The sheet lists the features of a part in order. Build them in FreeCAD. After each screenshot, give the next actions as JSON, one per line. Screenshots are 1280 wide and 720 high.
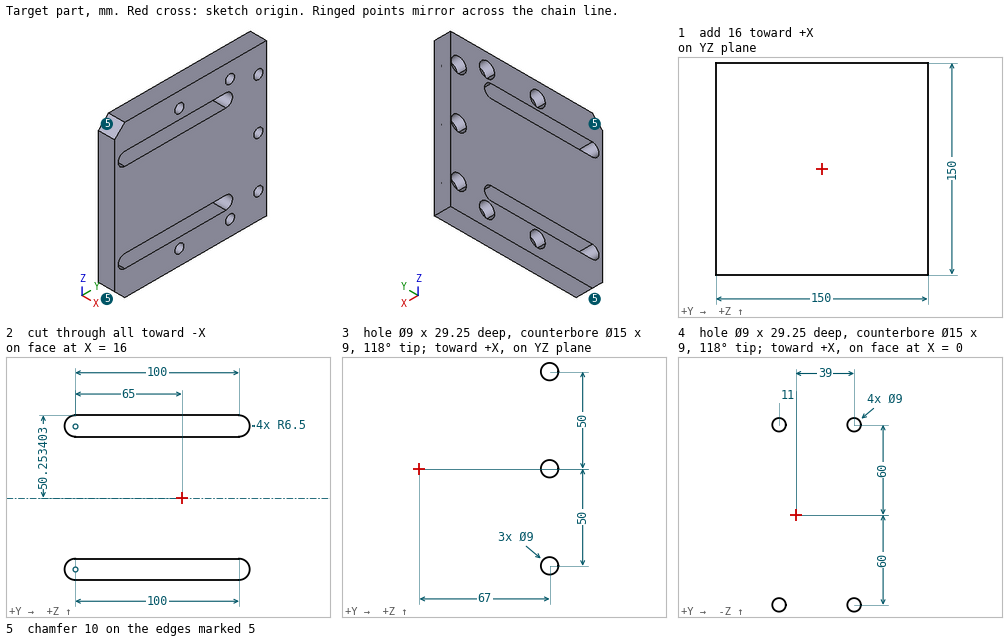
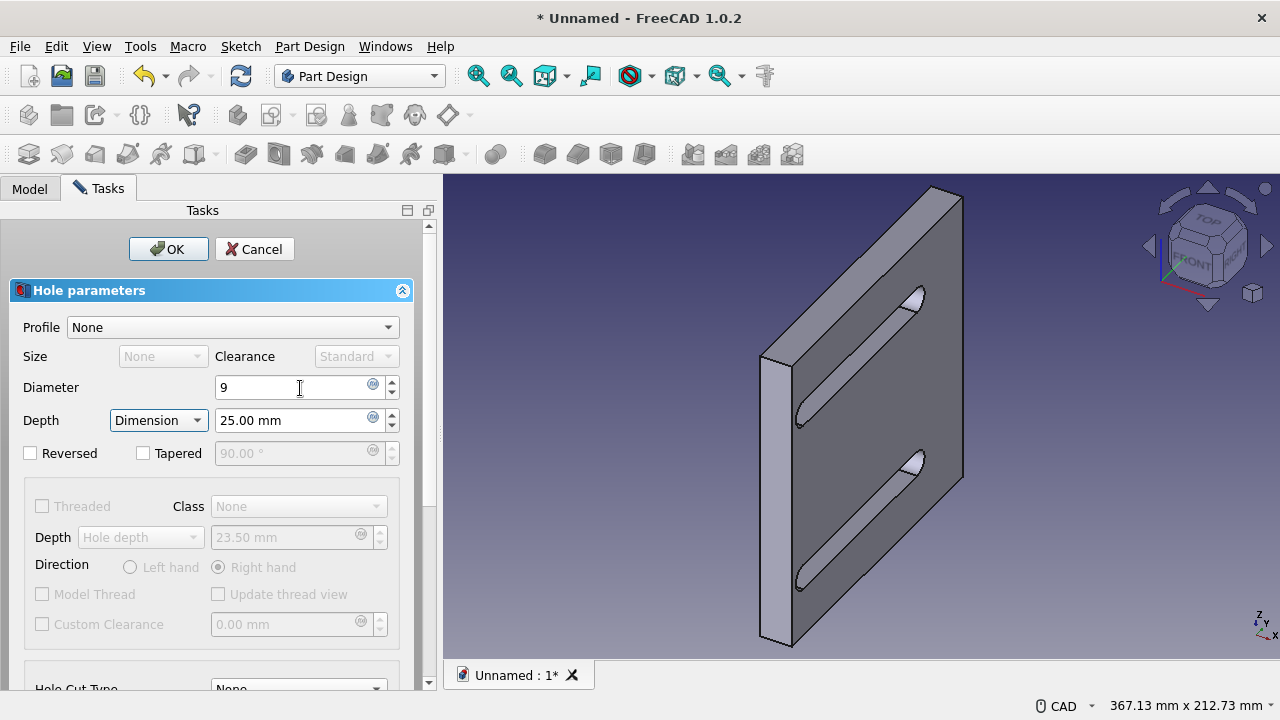
{"action": "triple_click", "coordinate": [300, 420]}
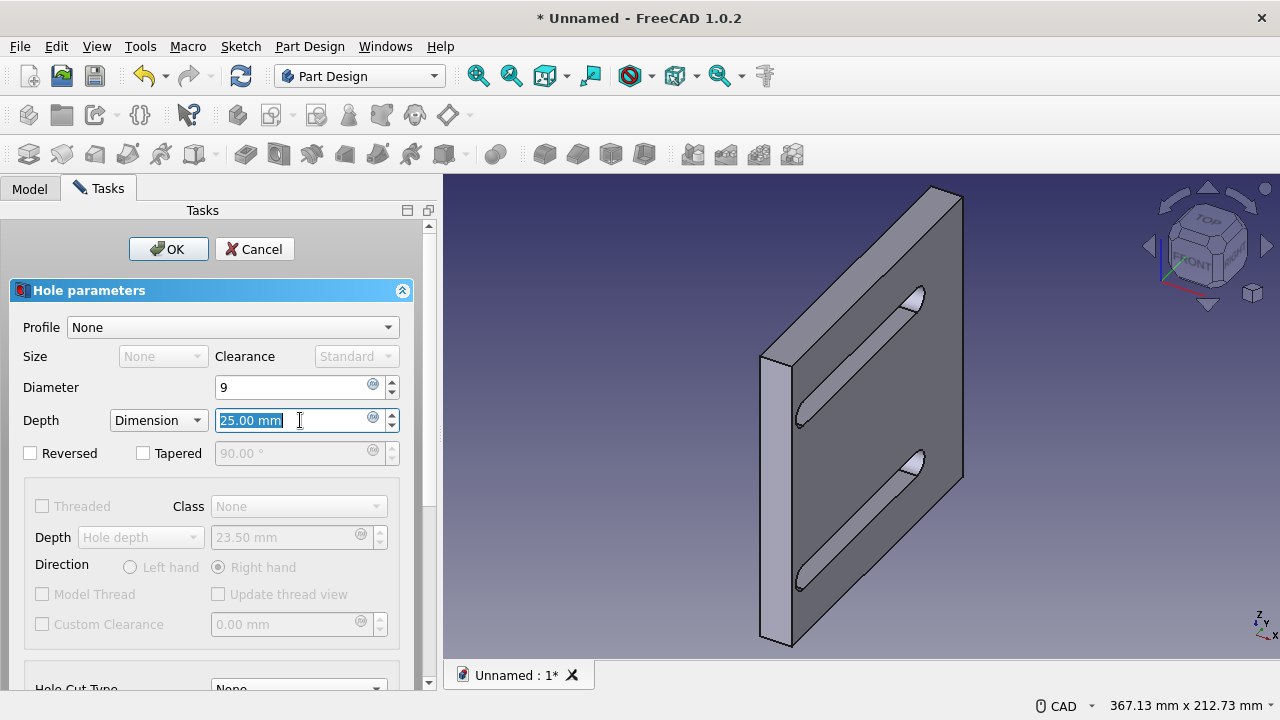
{"action": "type", "text": "29.25"}
{"action": "key", "text": "Tab"}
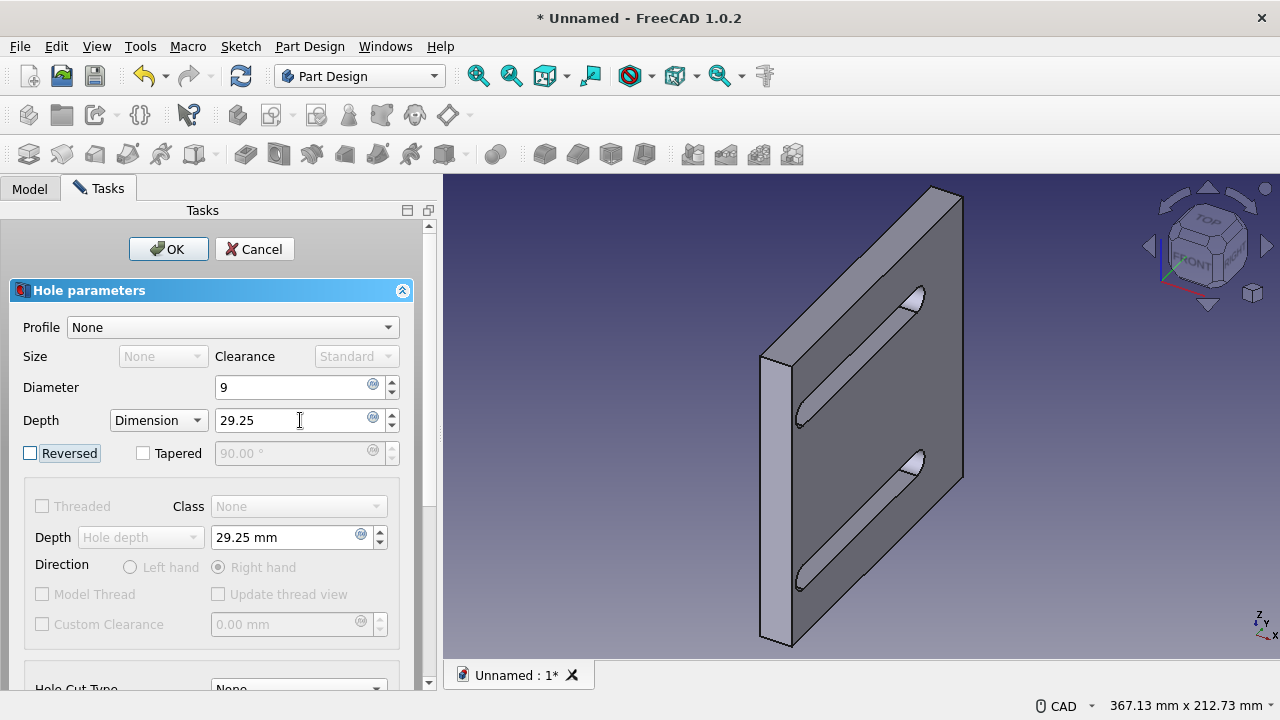
{"action": "left_click", "coordinate": [31, 453]}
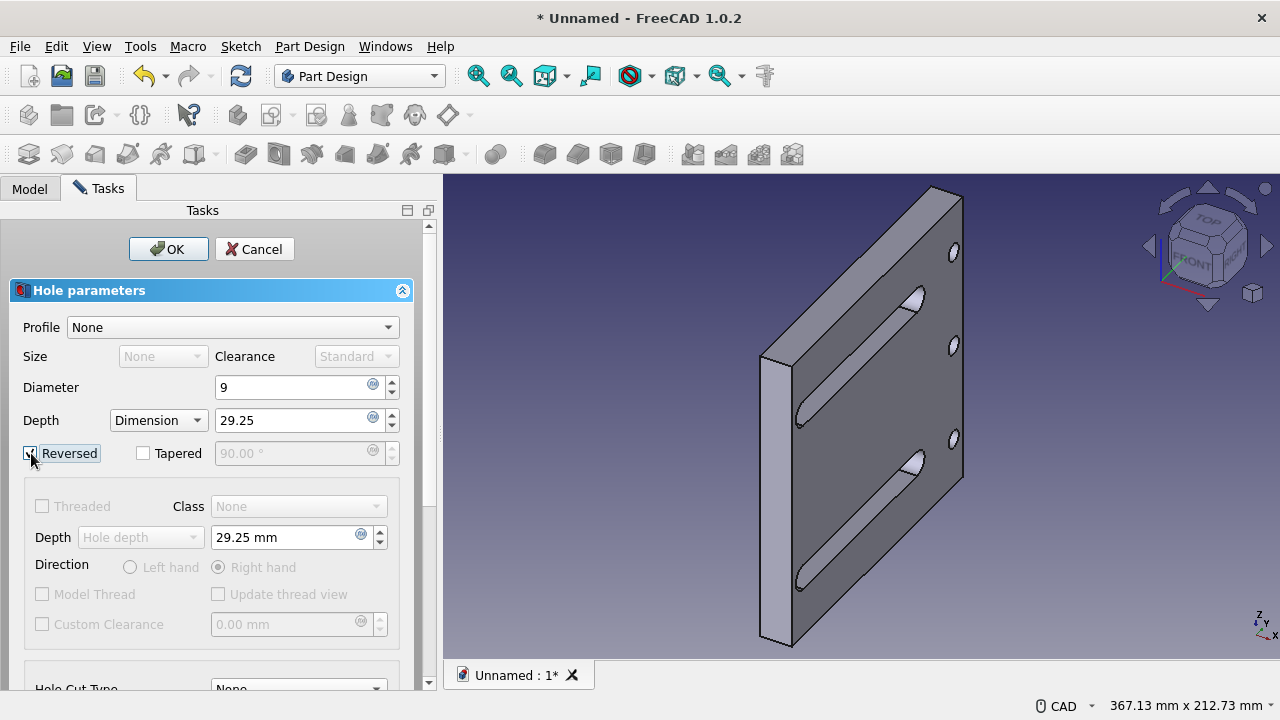
{"action": "scroll", "coordinate": [429, 455], "scroll_direction": "down", "scroll_amount": 2}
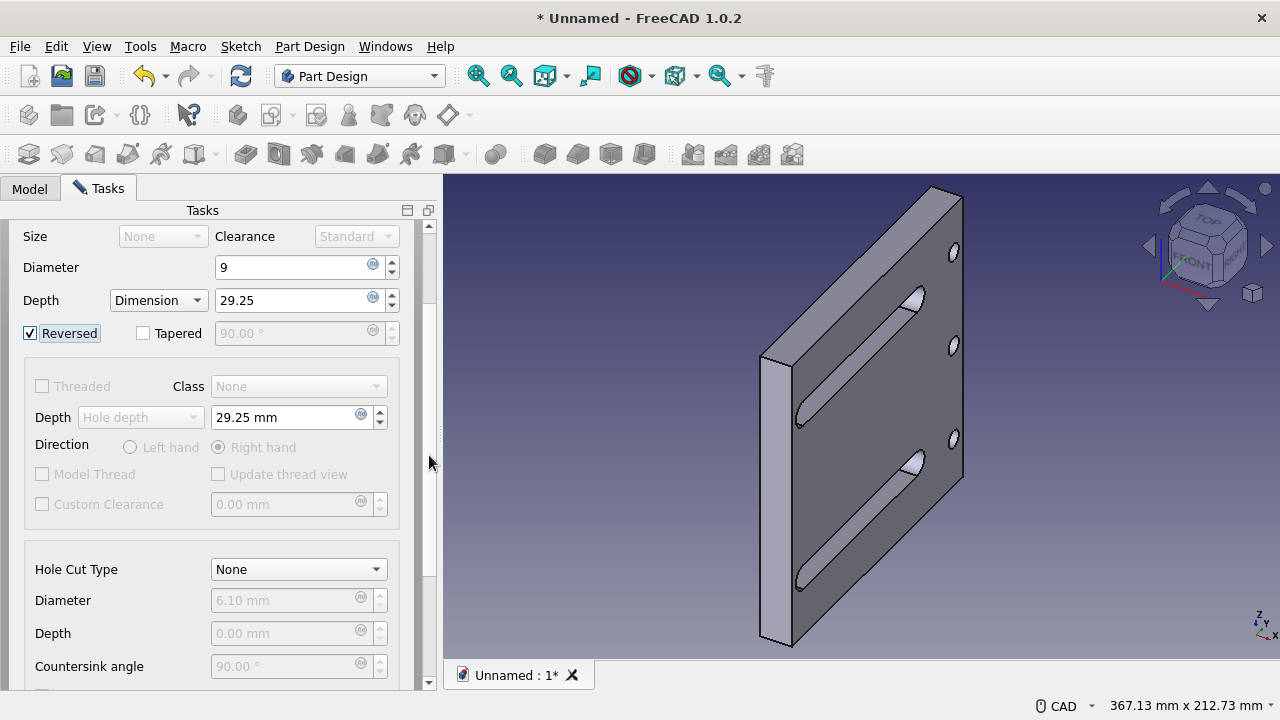
{"action": "left_click", "coordinate": [300, 570]}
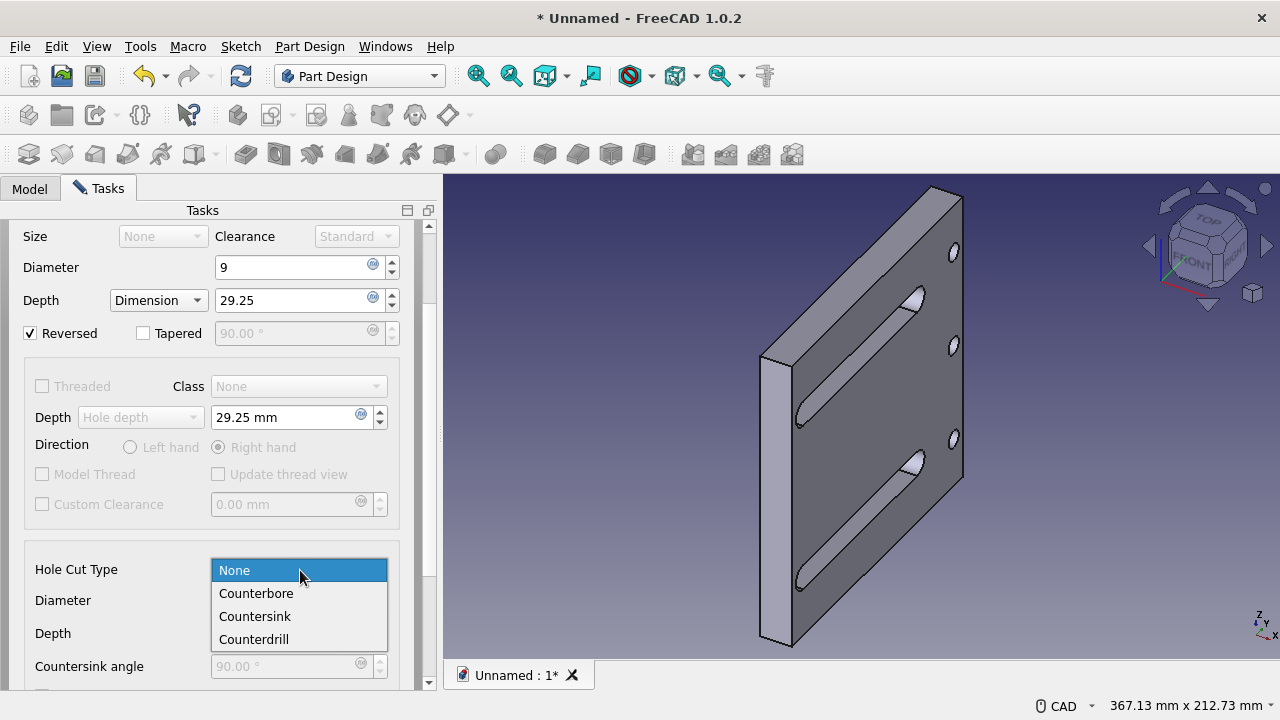
{"action": "left_click", "coordinate": [298, 594]}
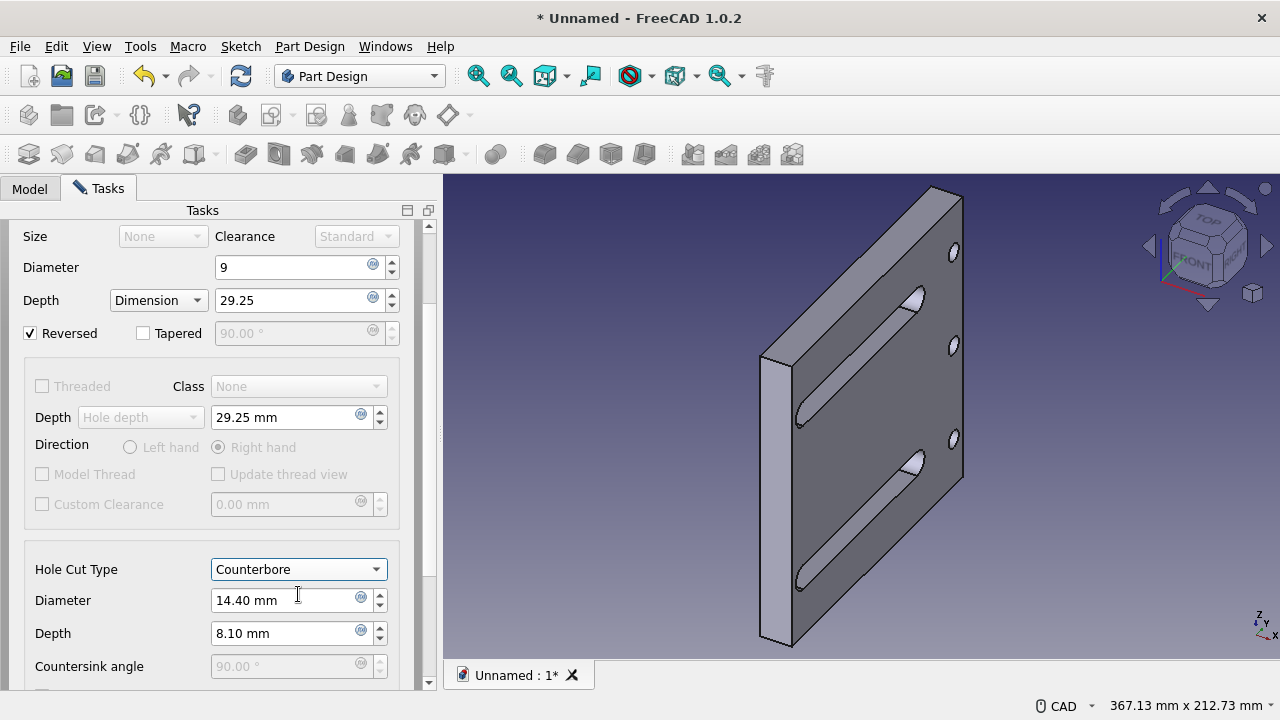
{"action": "triple_click", "coordinate": [292, 600]}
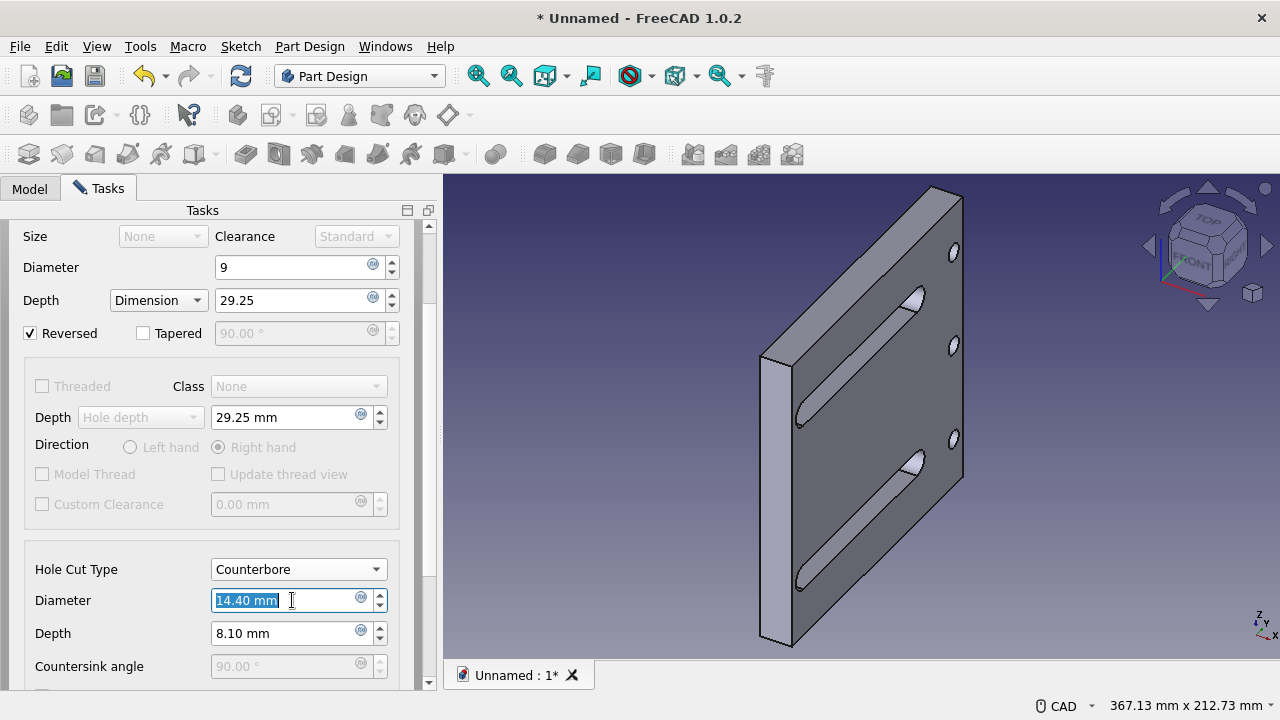
{"action": "type", "text": "15"}
{"action": "key", "text": "Tab"}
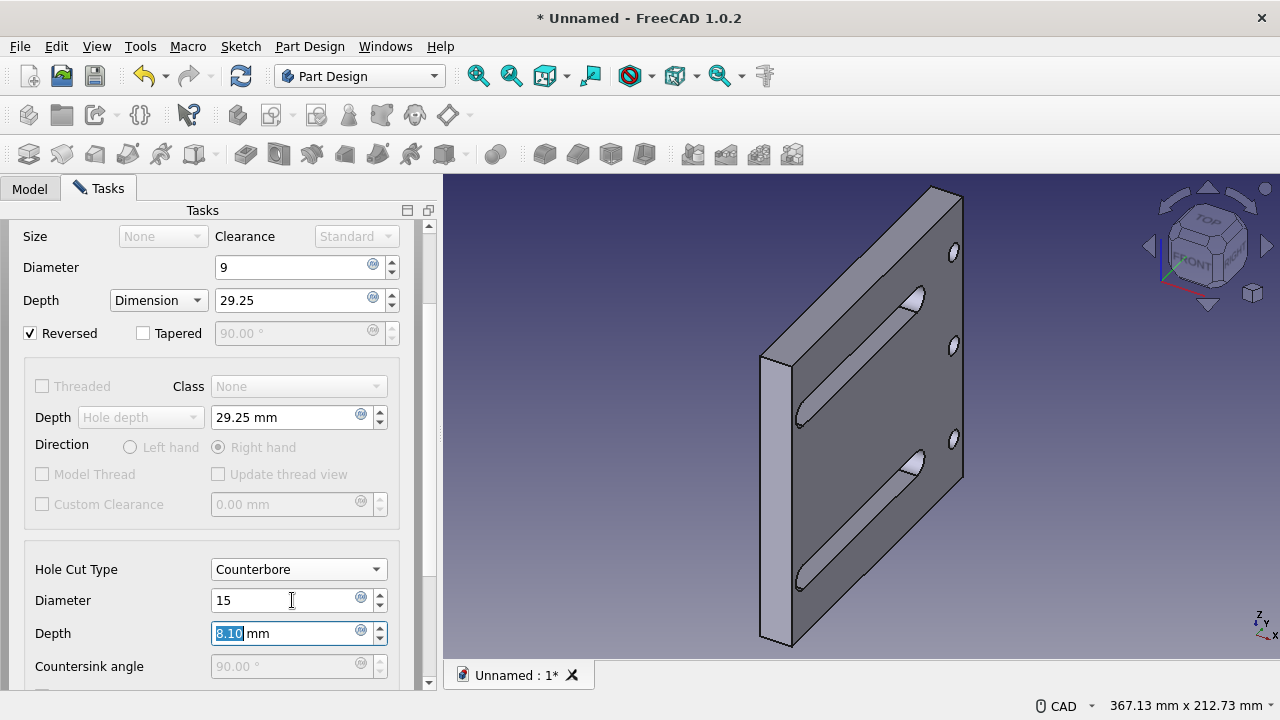
{"action": "type", "text": "9"}
{"action": "key", "text": "Tab"}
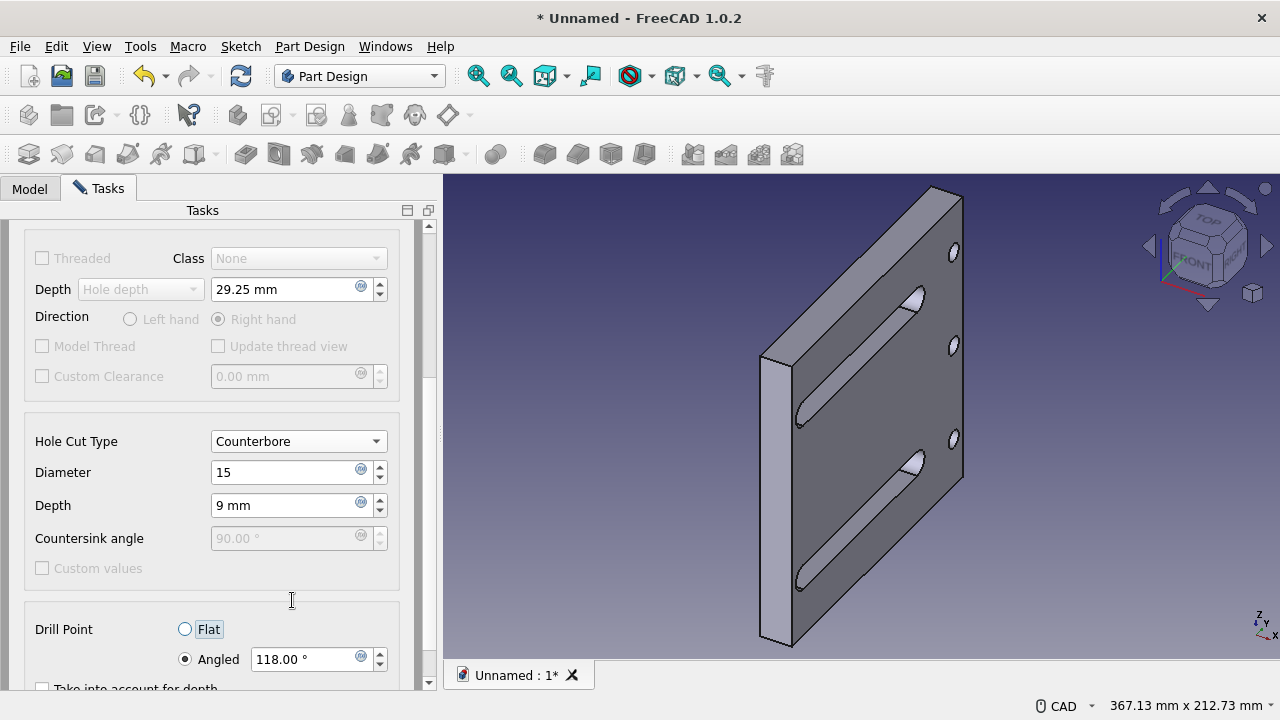
{"action": "scroll", "coordinate": [429, 455], "scroll_direction": "up", "scroll_amount": 5}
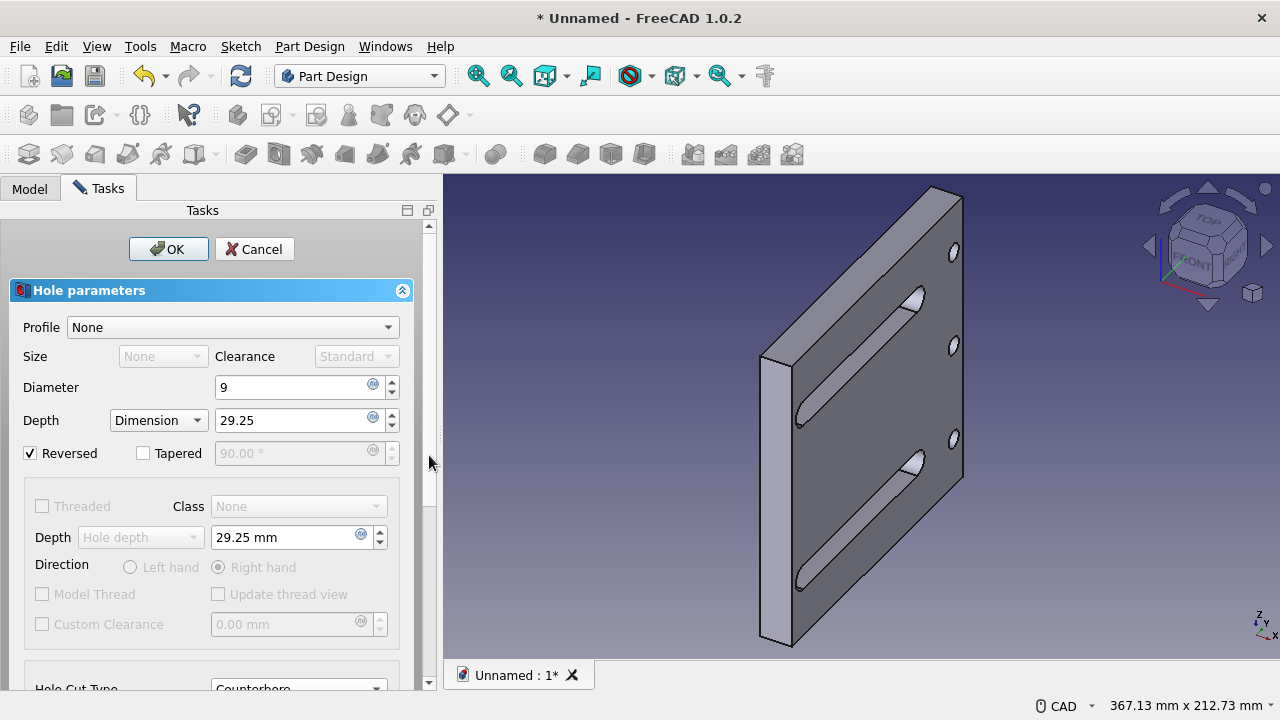
{"action": "left_click", "coordinate": [169, 249]}